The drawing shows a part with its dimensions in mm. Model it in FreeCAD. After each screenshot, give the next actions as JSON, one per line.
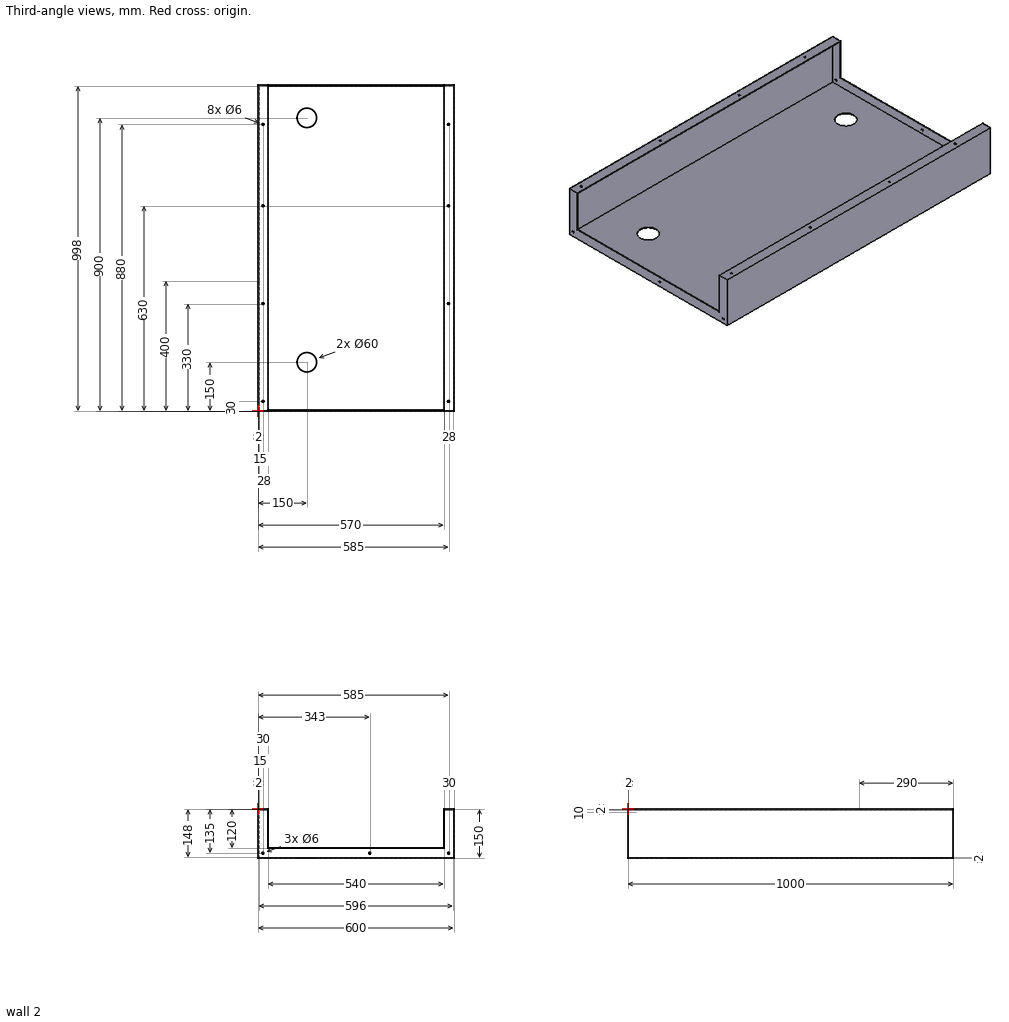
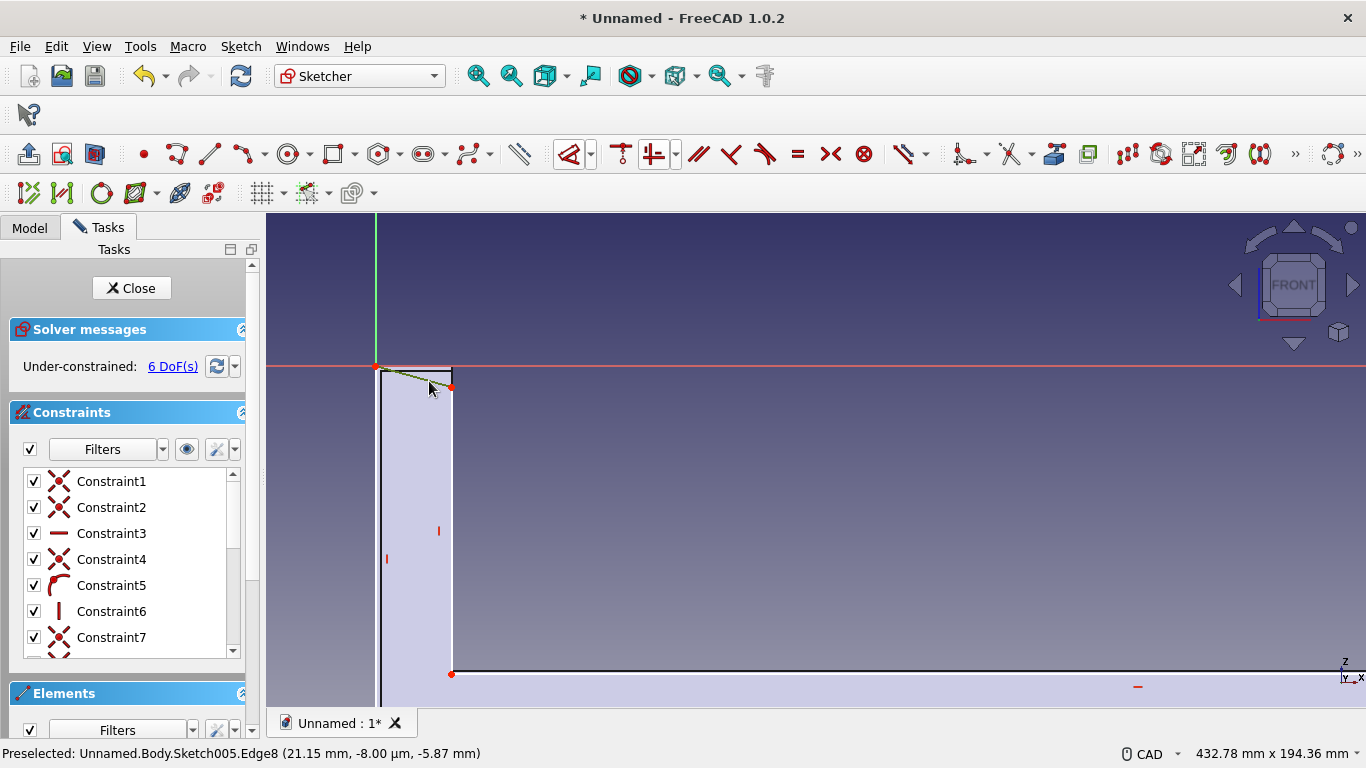
{"action": "key", "text": "h"}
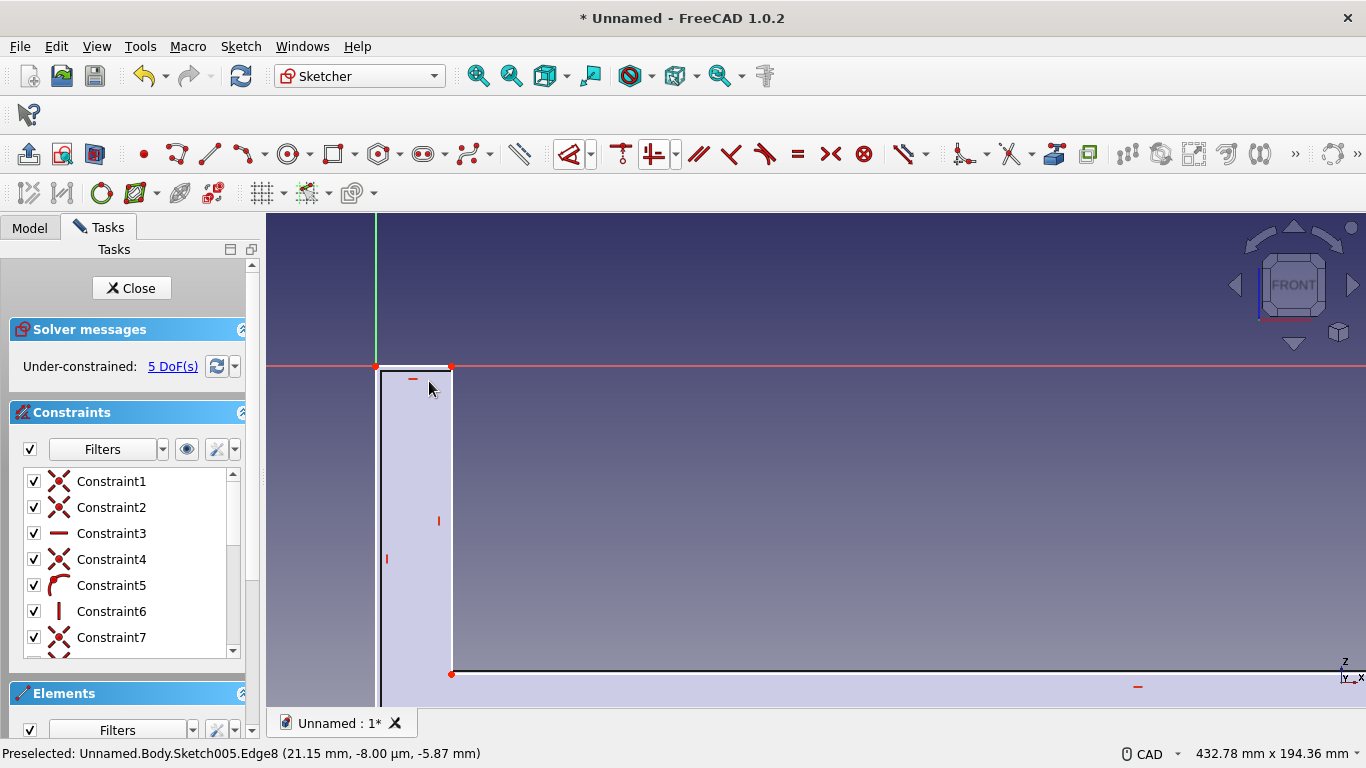
{"action": "scroll", "coordinate": [429, 381], "scroll_direction": "down", "scroll_amount": 4}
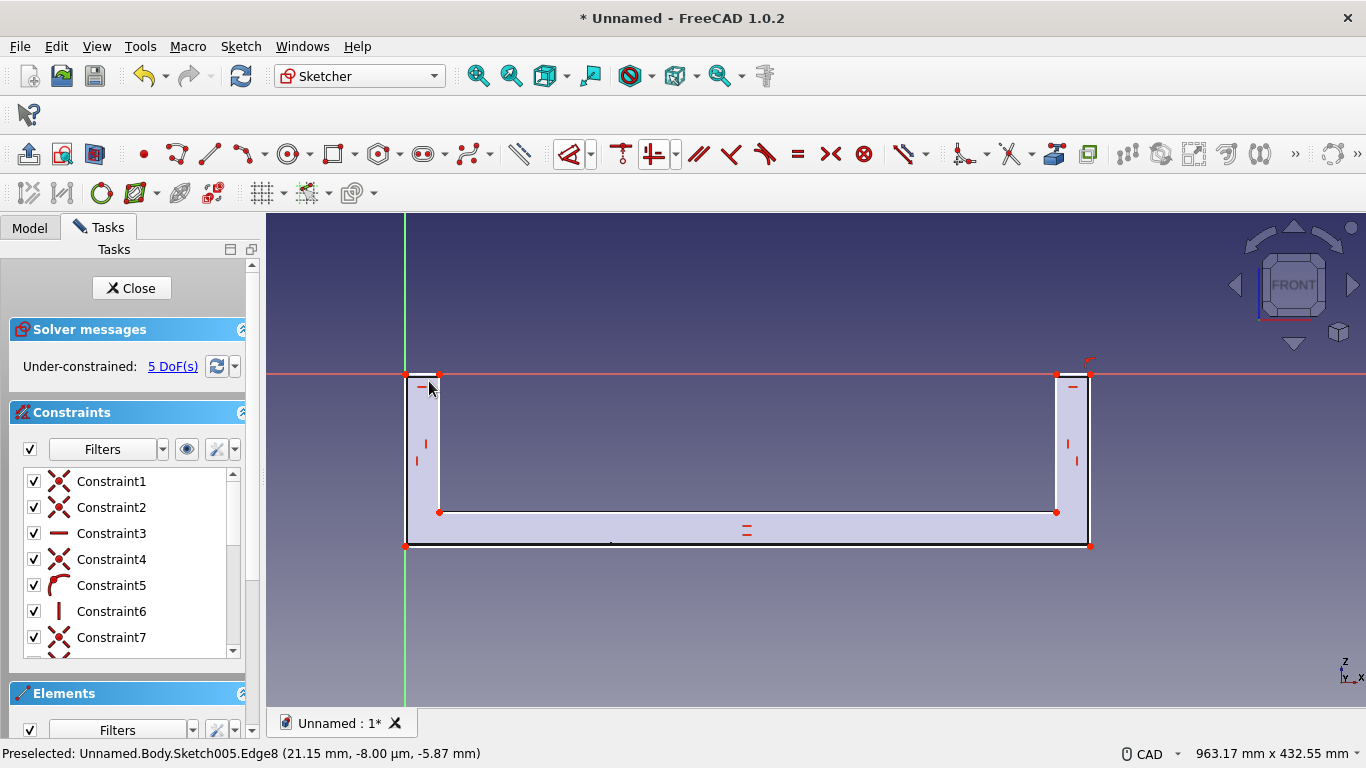
{"action": "scroll", "coordinate": [1080, 374], "scroll_direction": "up", "scroll_amount": 2}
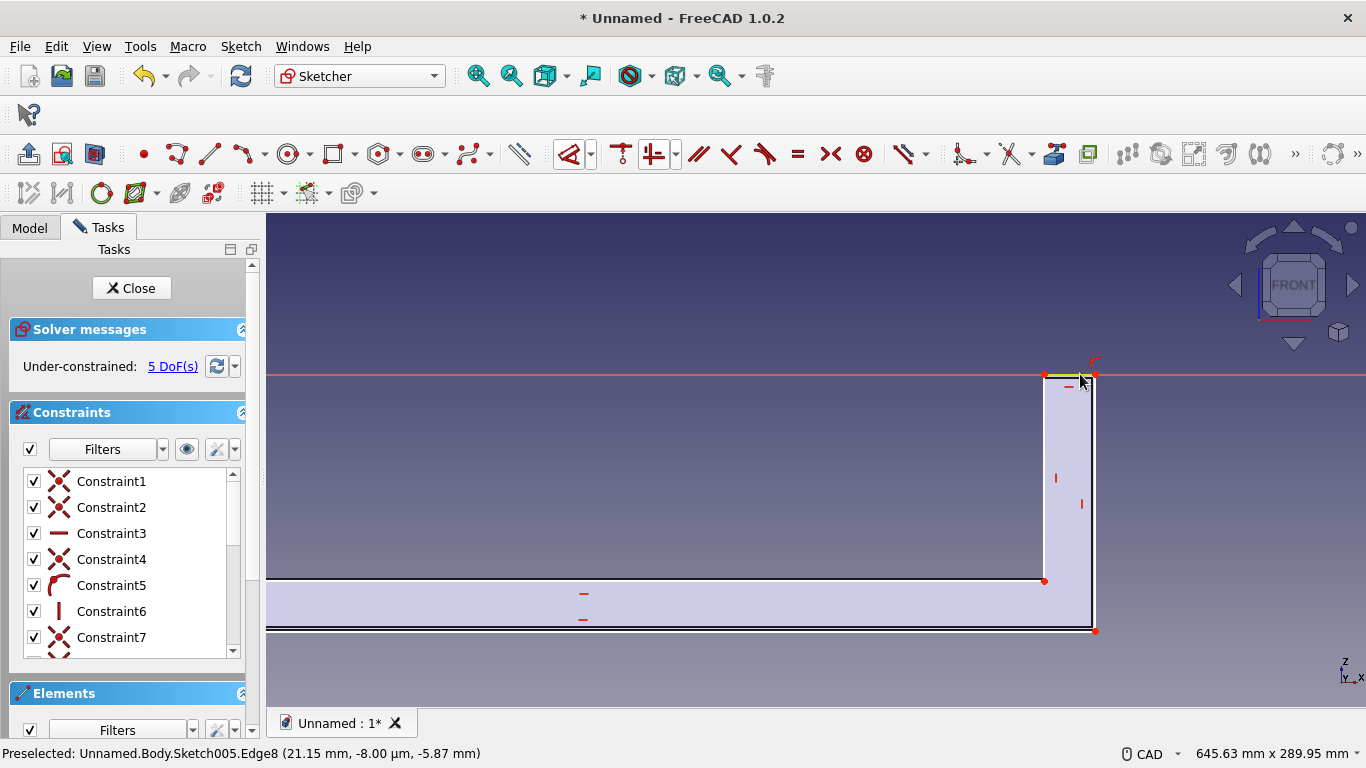
{"action": "left_click", "coordinate": [1080, 375]}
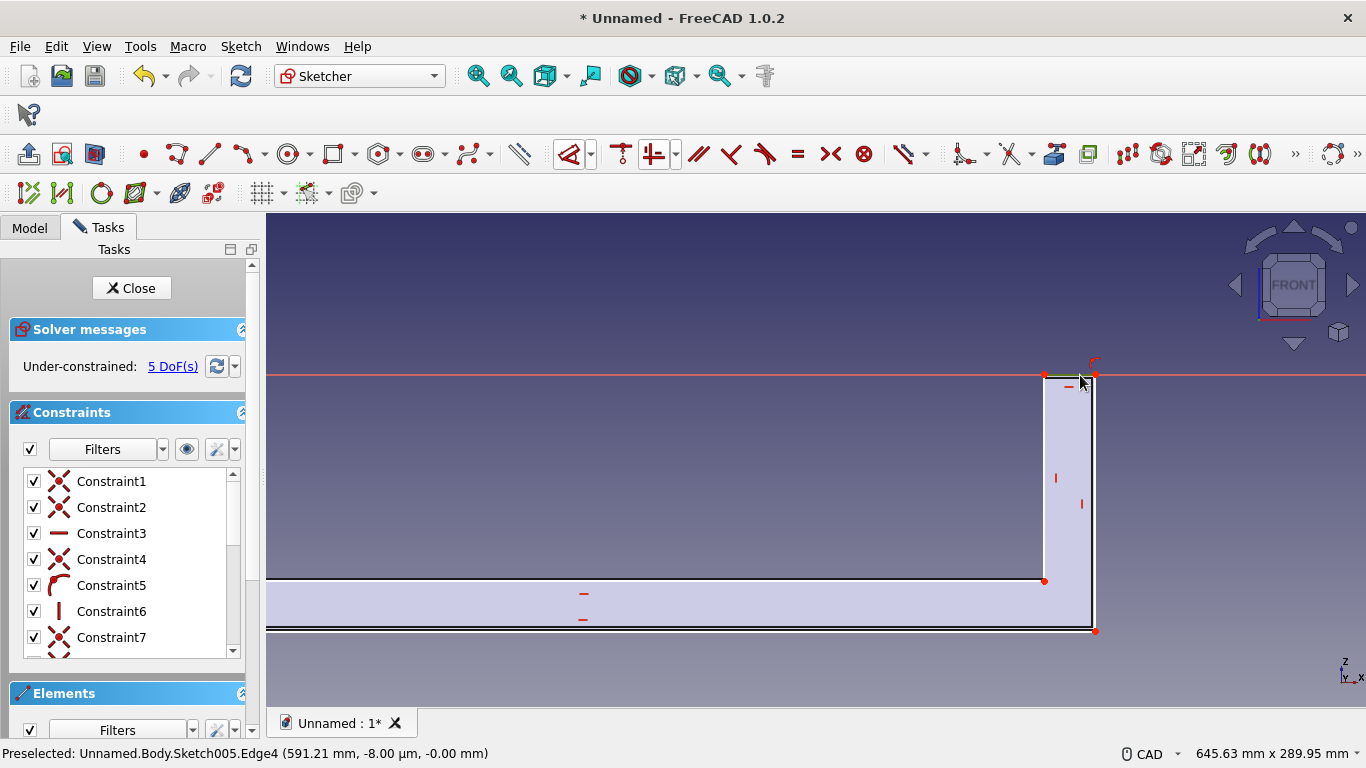
{"action": "key", "text": "l"}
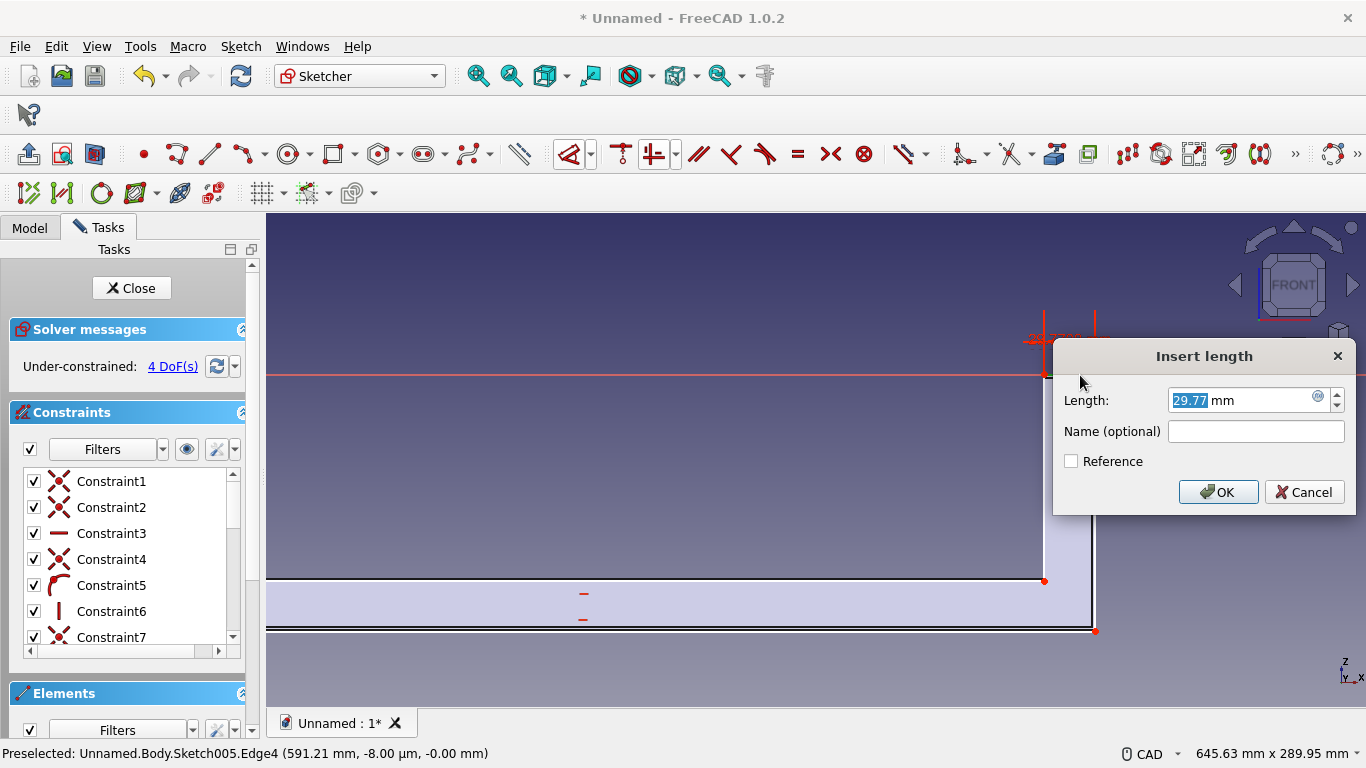
{"action": "type", "text": "30"}
{"action": "key", "text": "Return"}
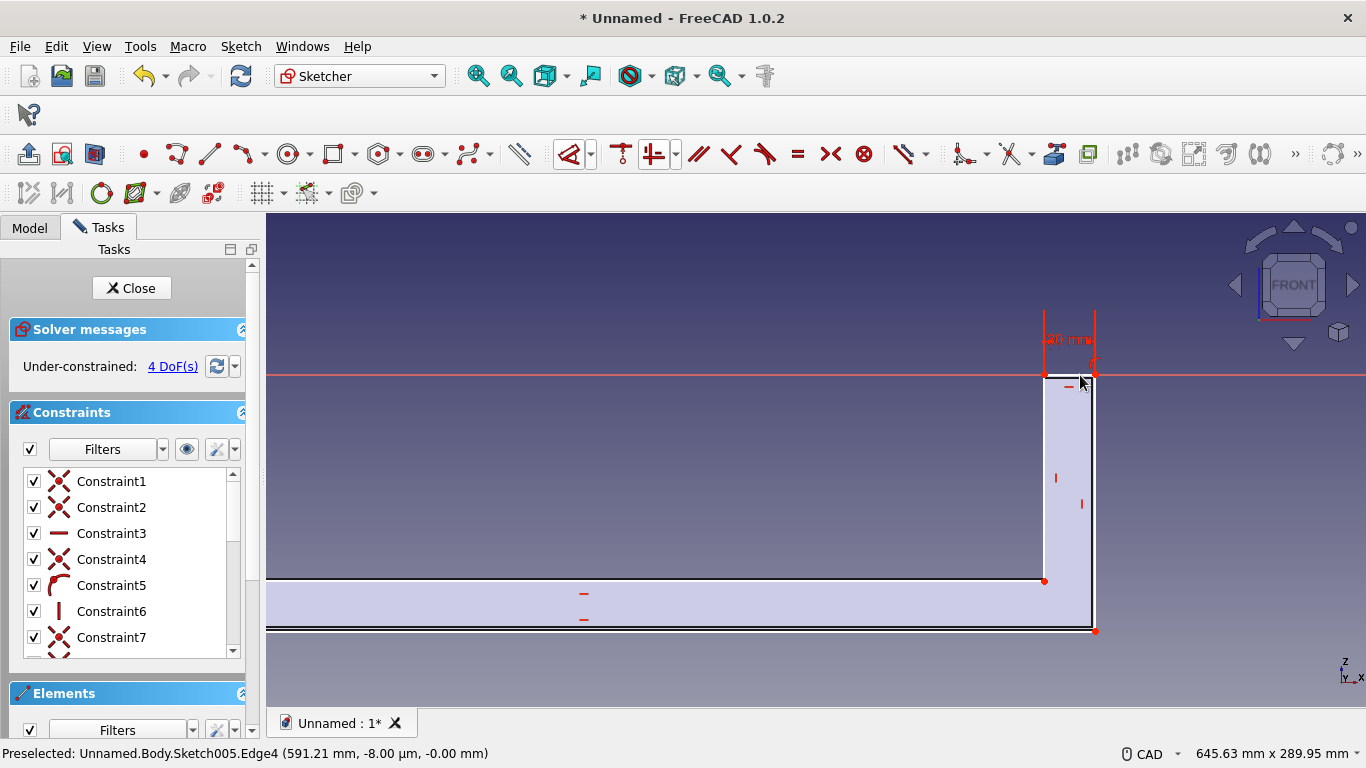
{"action": "scroll", "coordinate": [1080, 374], "scroll_direction": "down", "scroll_amount": 2}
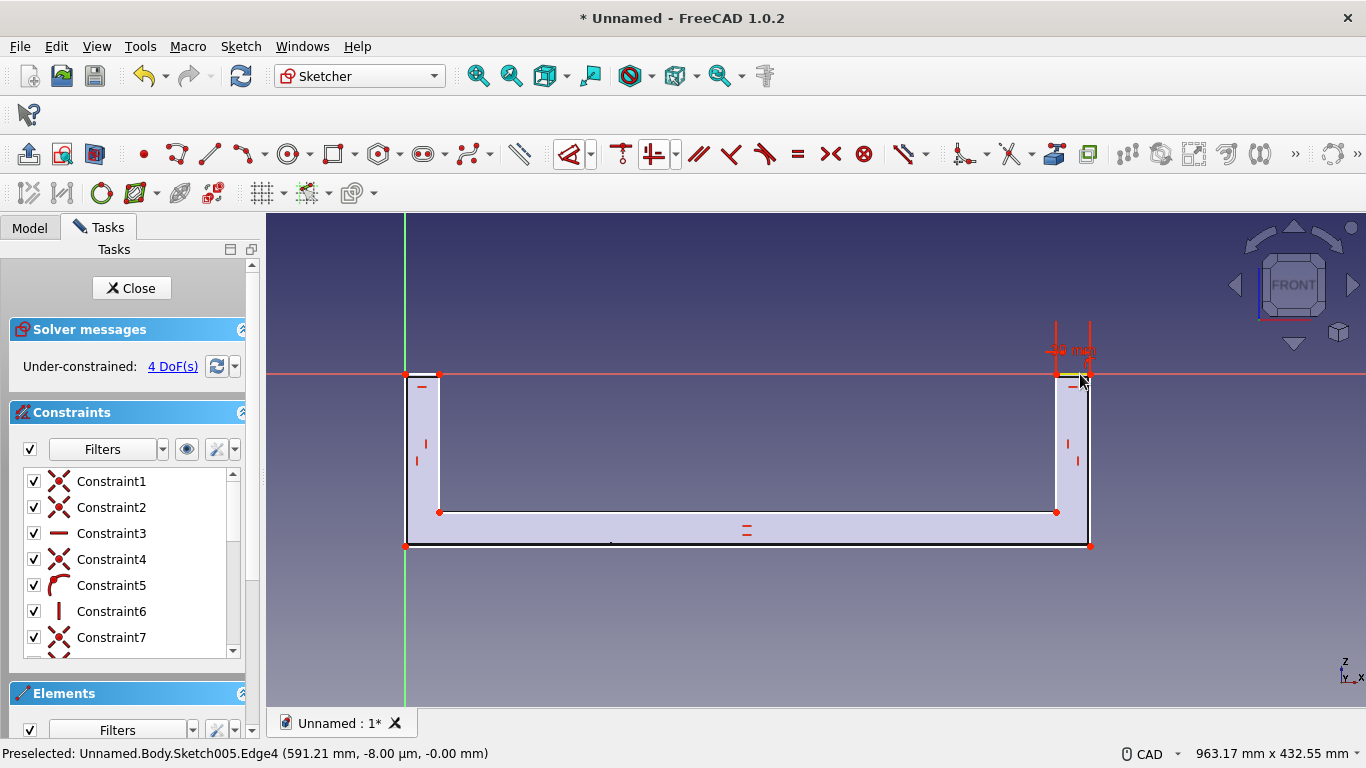
{"action": "scroll", "coordinate": [429, 374], "scroll_direction": "up", "scroll_amount": 2}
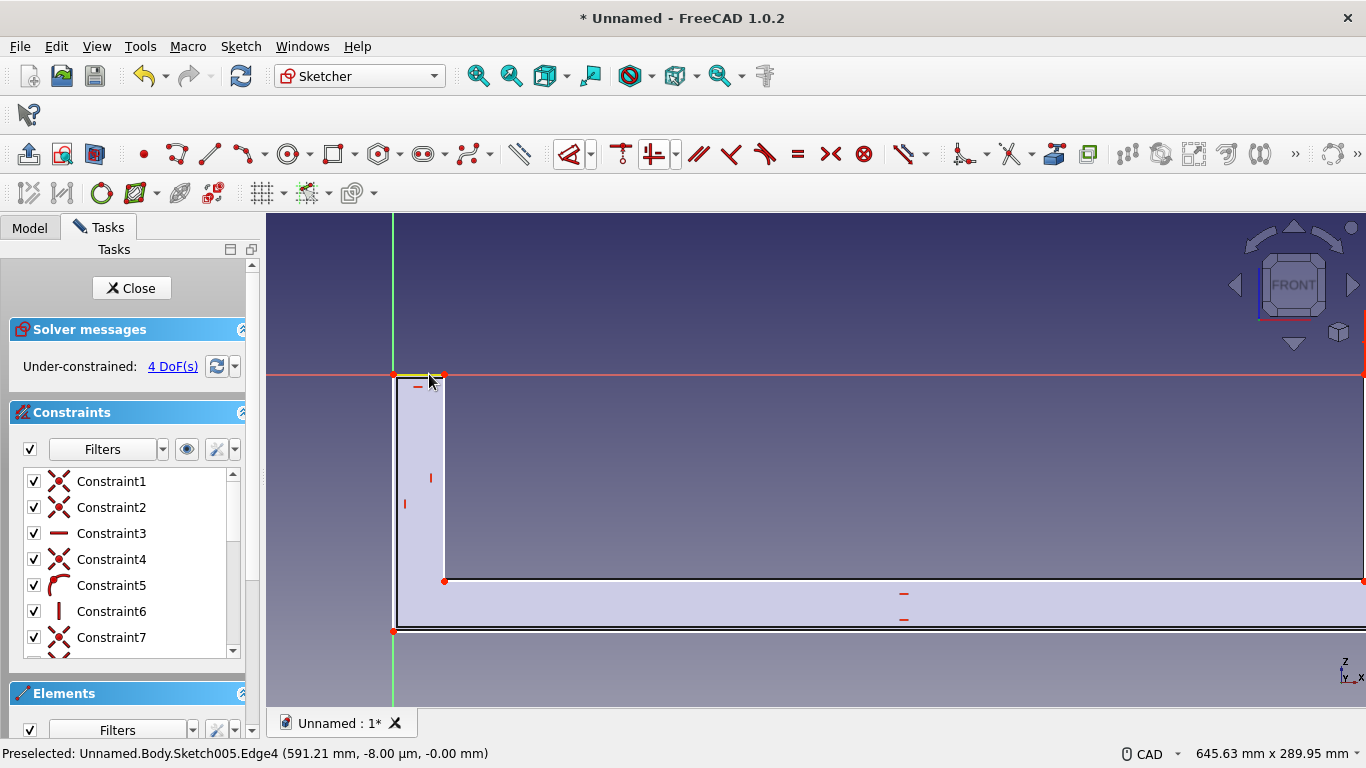
{"action": "left_click", "coordinate": [429, 375]}